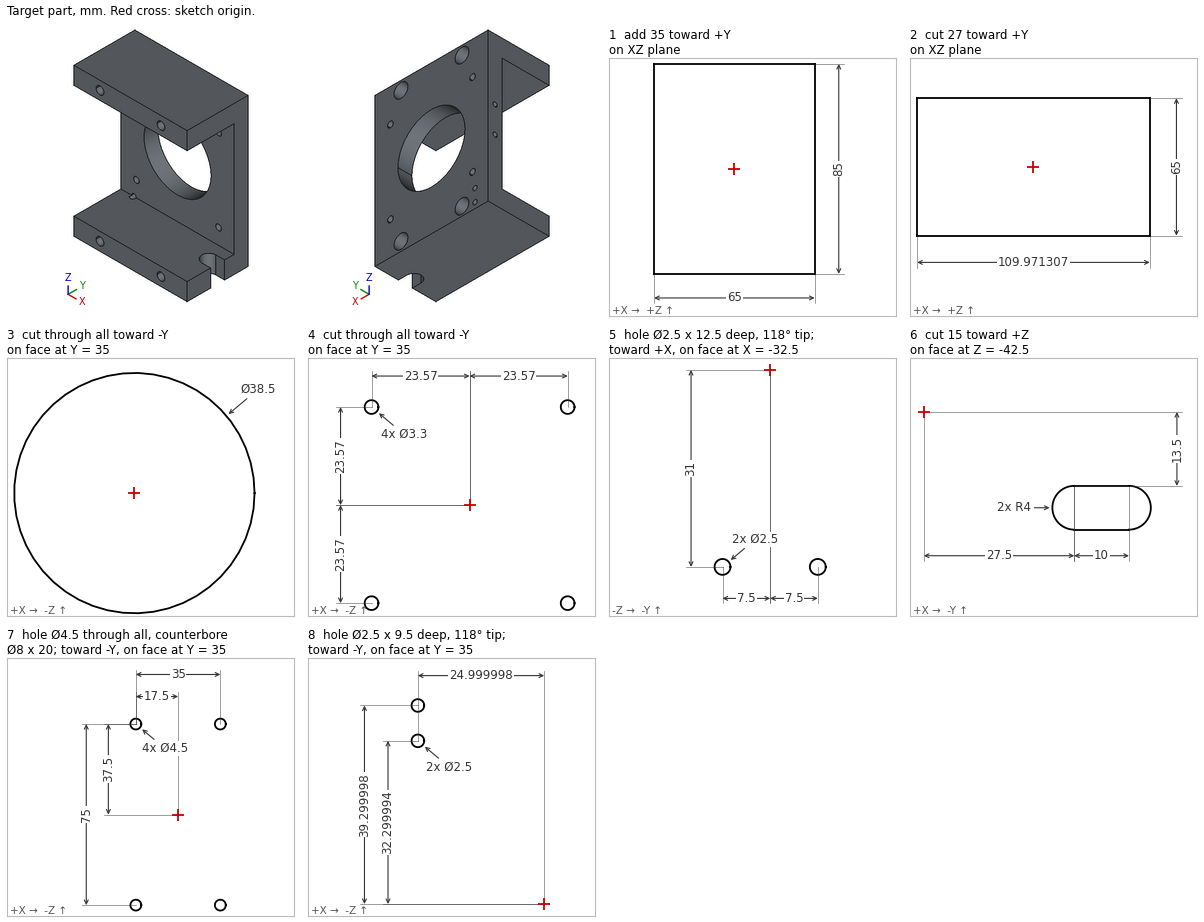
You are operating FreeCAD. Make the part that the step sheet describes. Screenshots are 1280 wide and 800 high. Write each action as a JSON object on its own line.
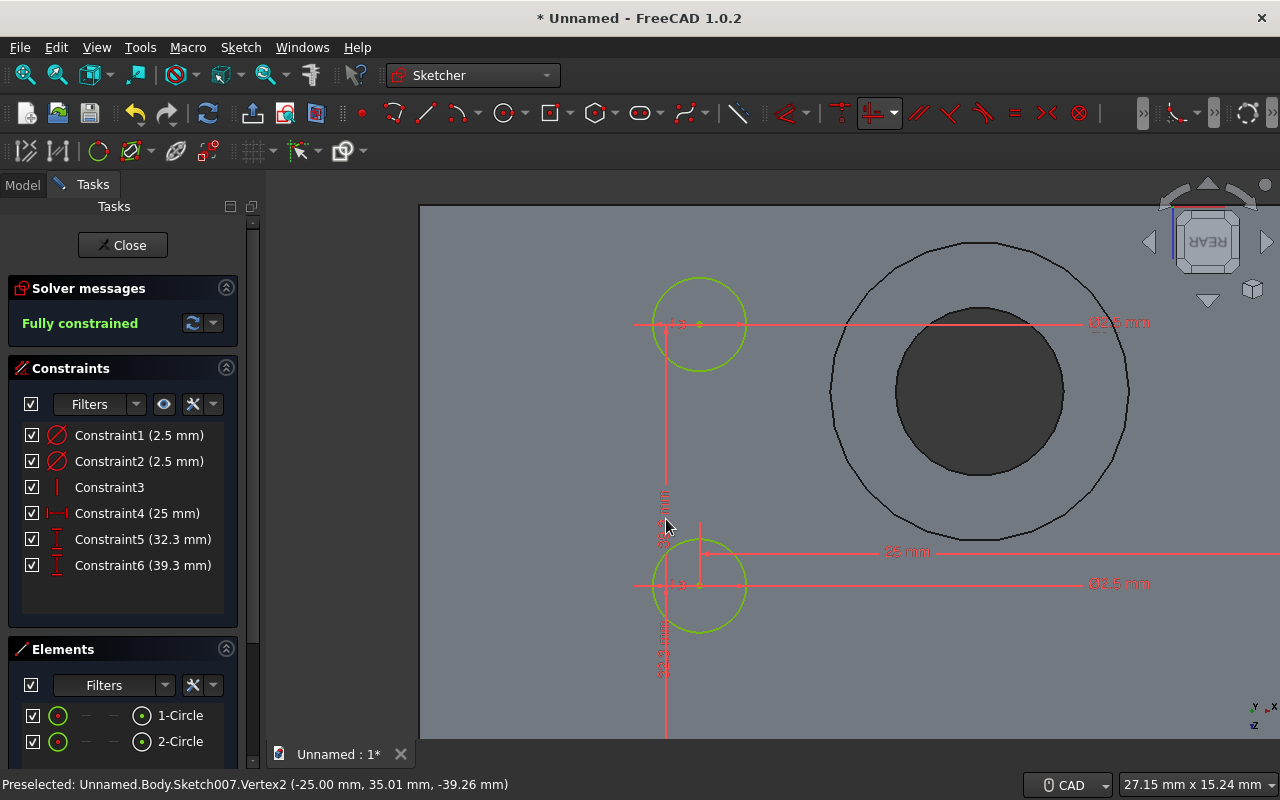
{"action": "left_click", "coordinate": [123, 245]}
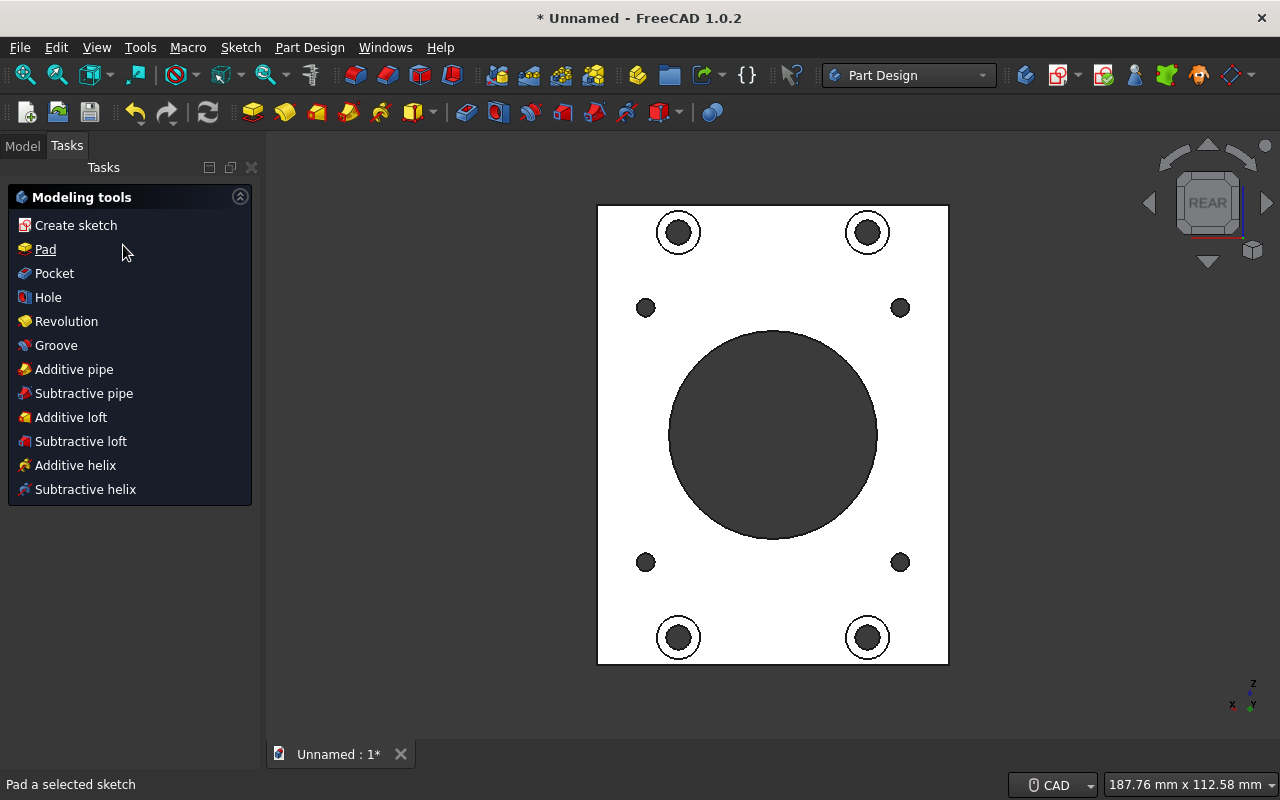
{"action": "left_click", "coordinate": [500, 112]}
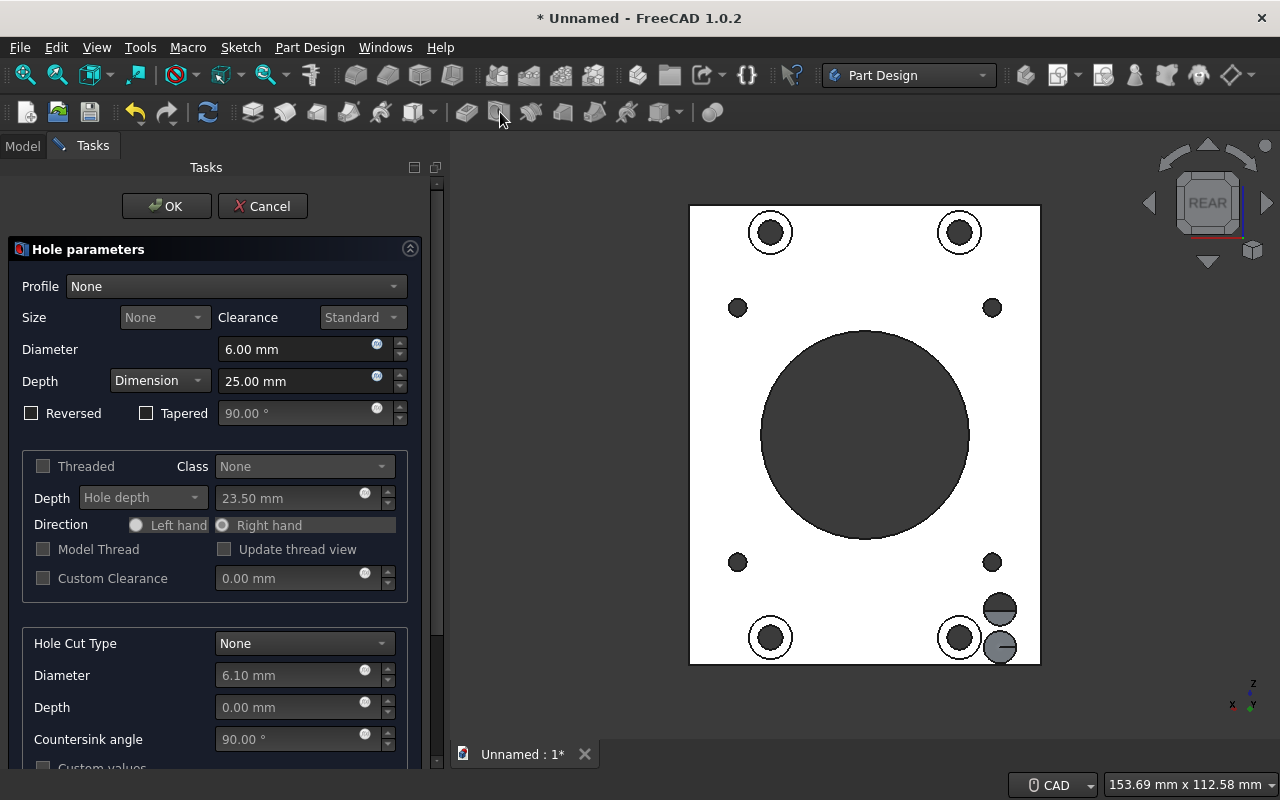
{"action": "triple_click", "coordinate": [305, 349]}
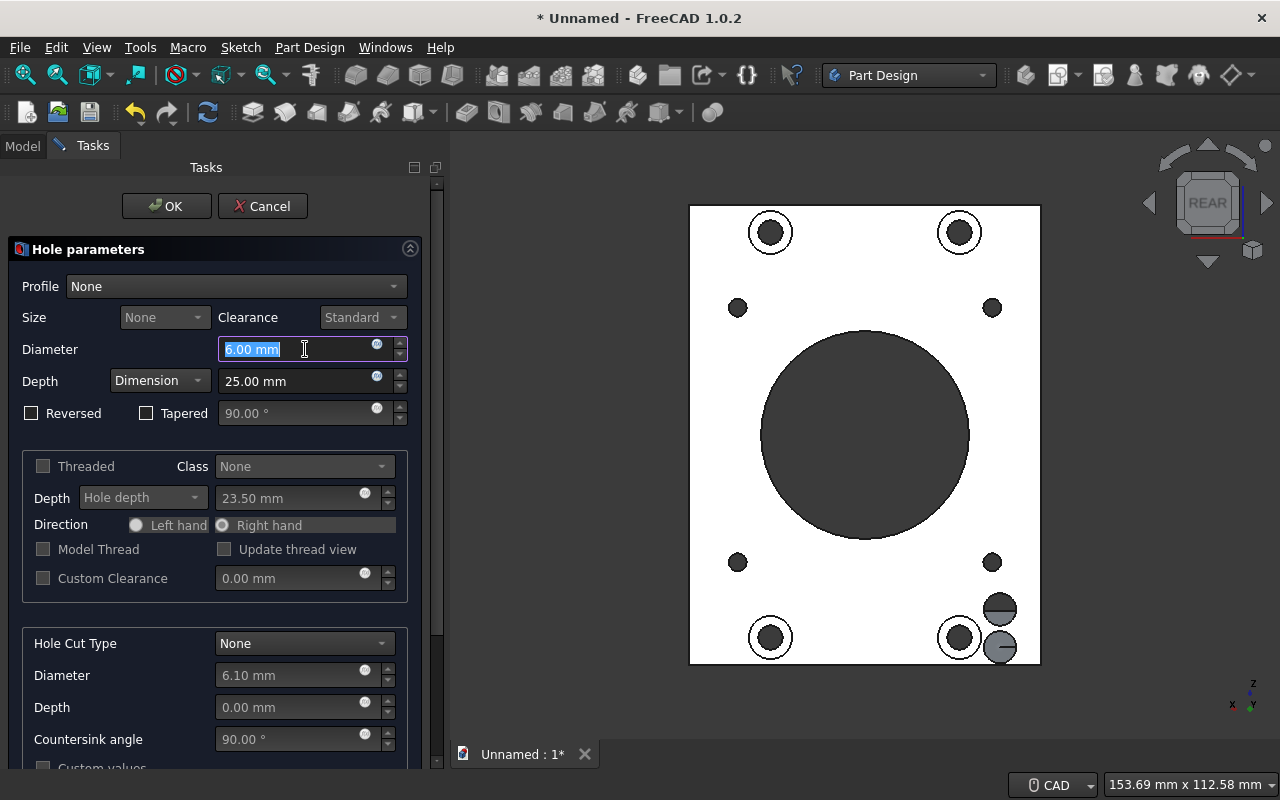
{"action": "type", "text": "2.5"}
{"action": "key", "text": "Tab"}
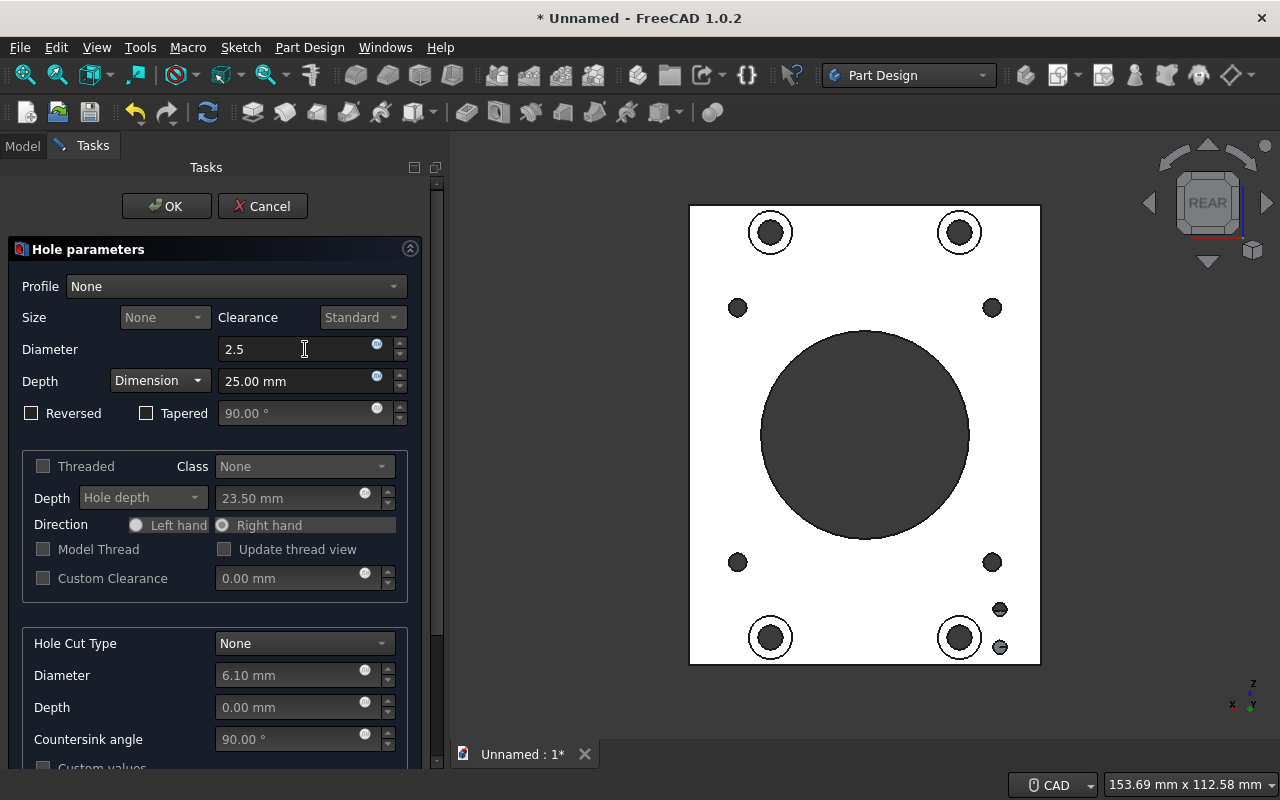
{"action": "triple_click", "coordinate": [305, 381]}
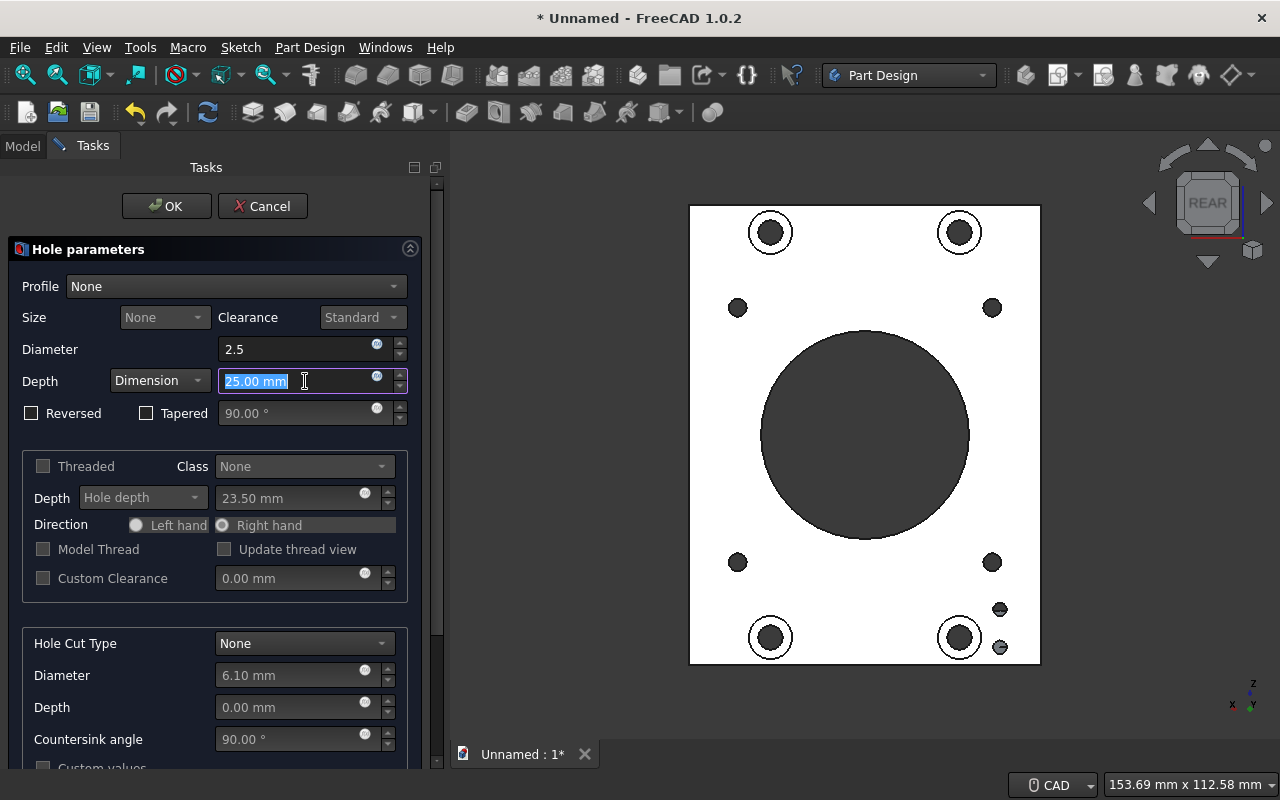
{"action": "type", "text": "9.5"}
{"action": "key", "text": "Tab"}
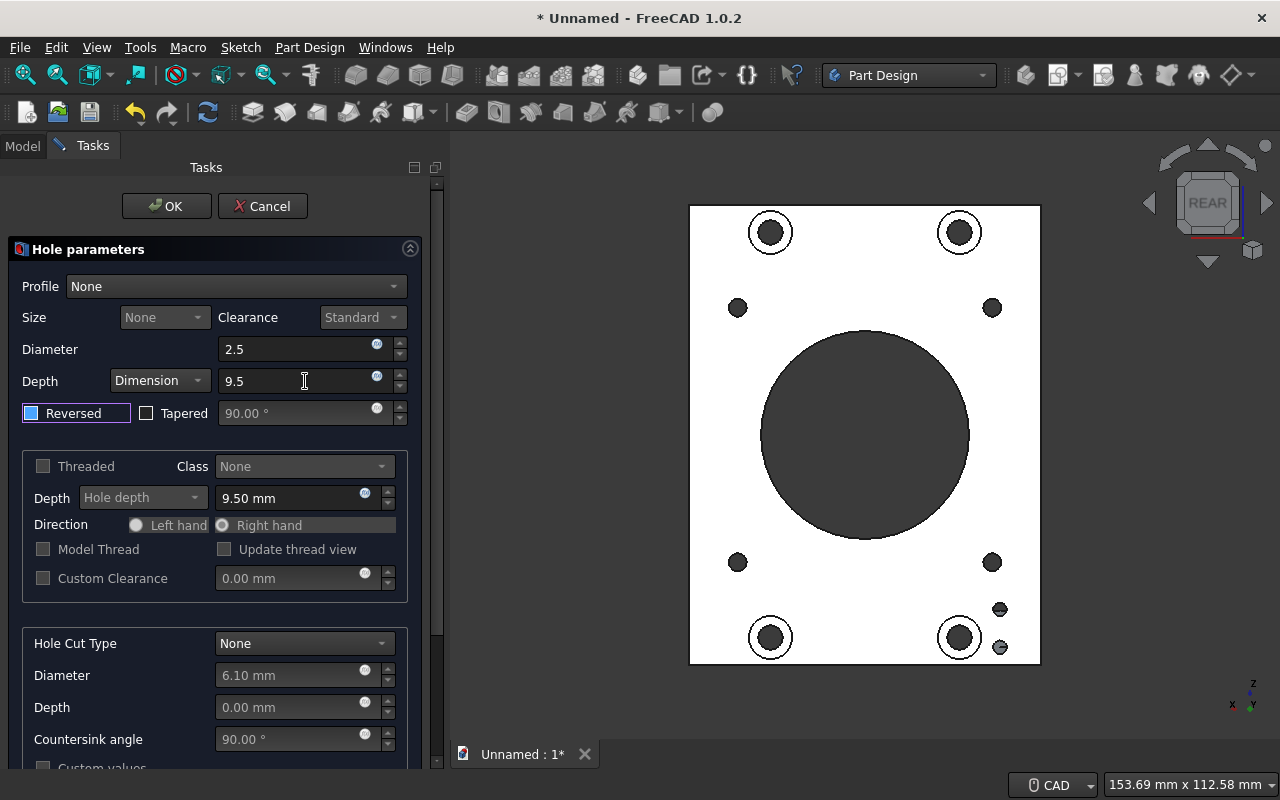
{"action": "left_click", "coordinate": [167, 206]}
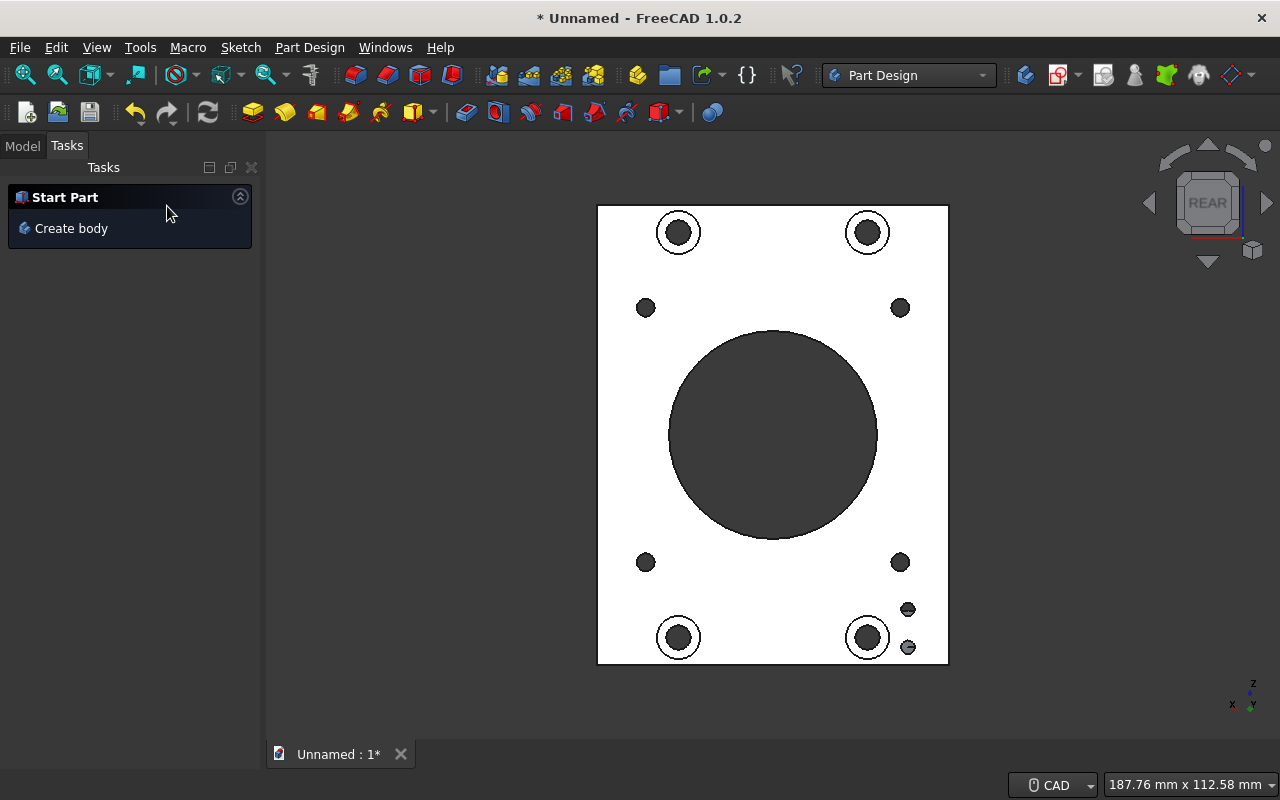
{"action": "key", "text": "0"}